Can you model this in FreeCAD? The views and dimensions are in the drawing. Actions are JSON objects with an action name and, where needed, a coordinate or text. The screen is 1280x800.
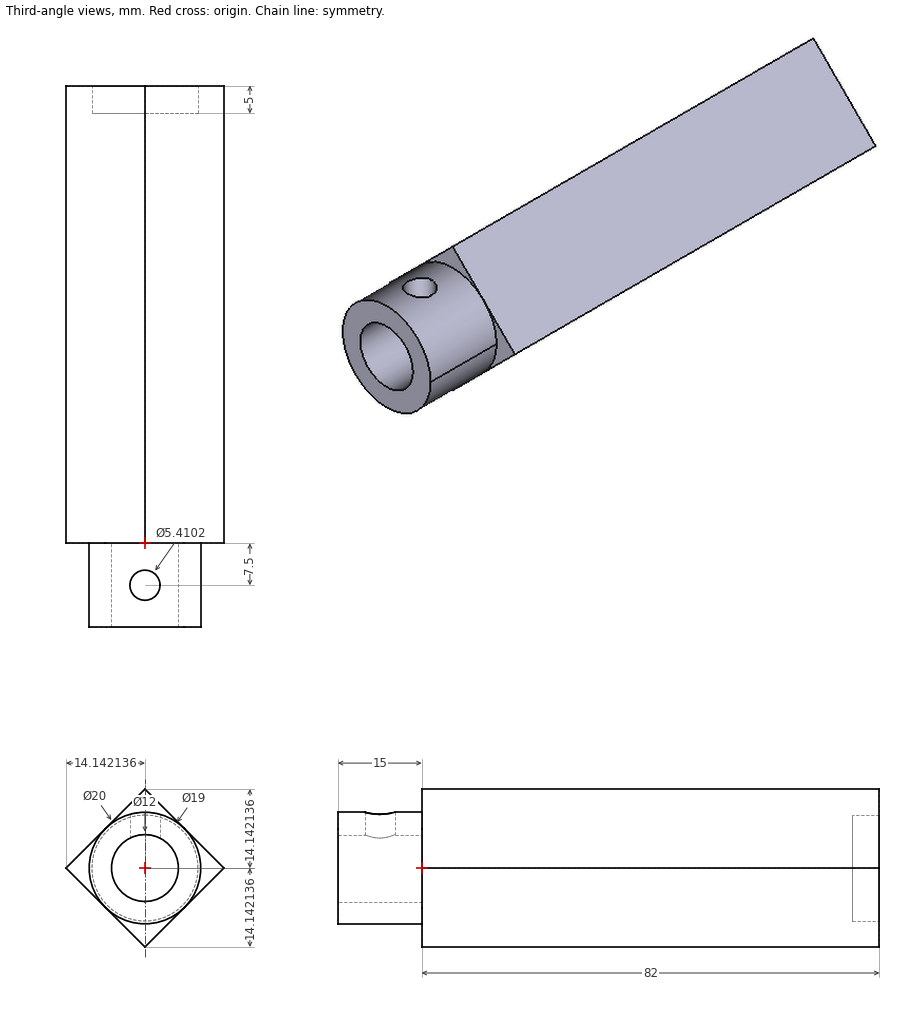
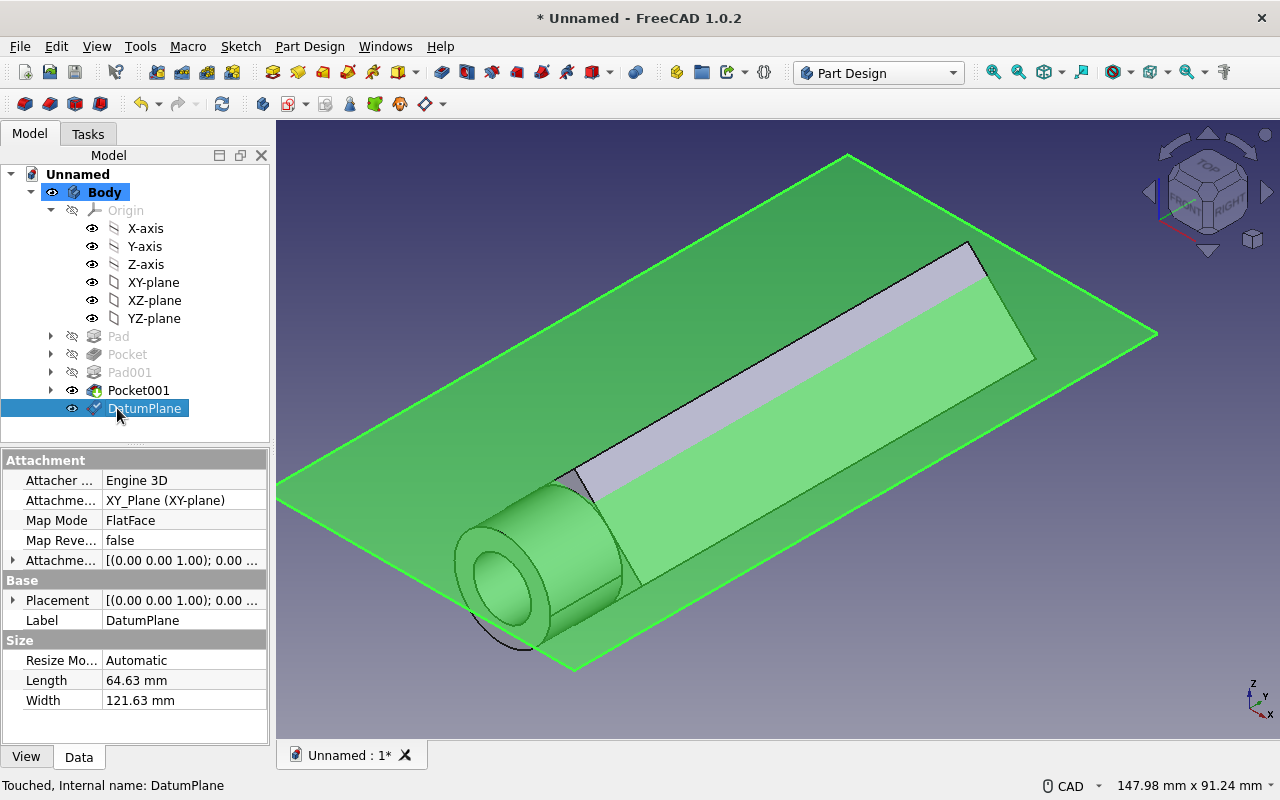
{"action": "left_click", "coordinate": [288, 104]}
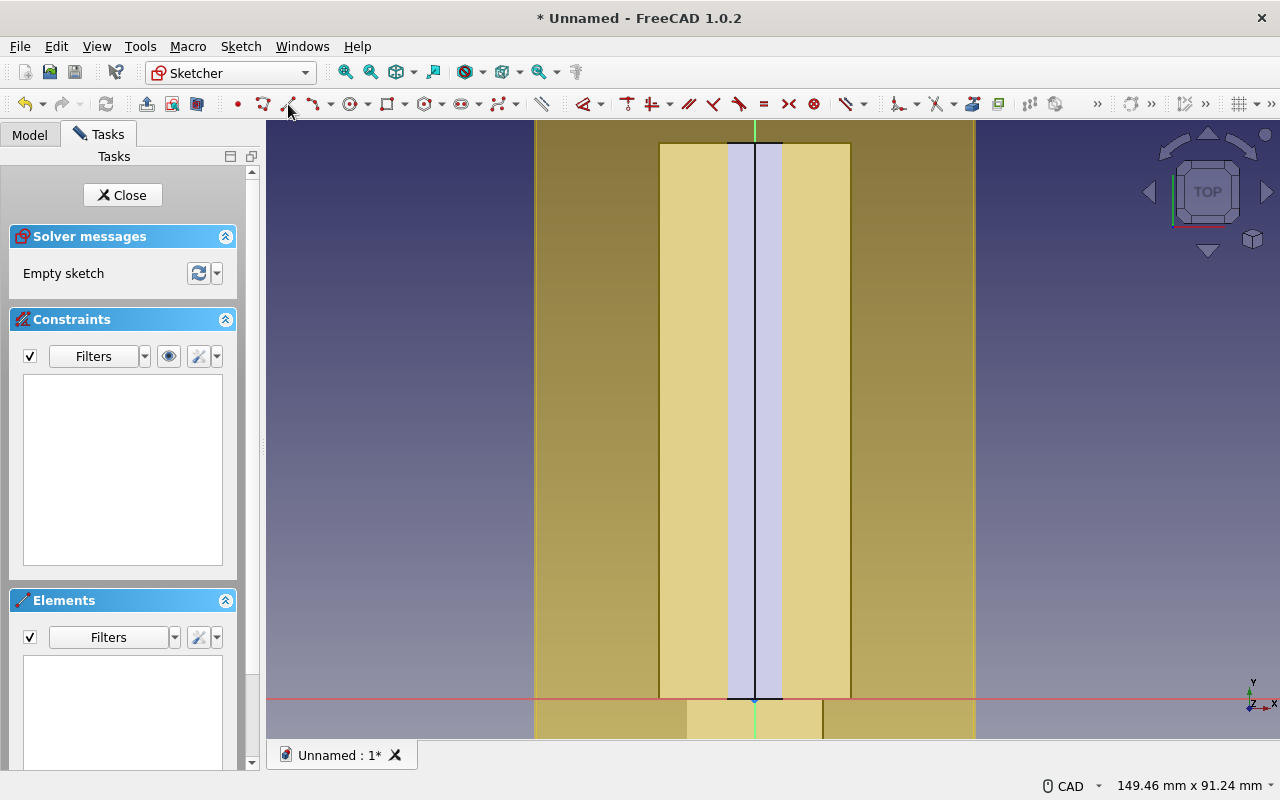
{"action": "key", "text": "q s"}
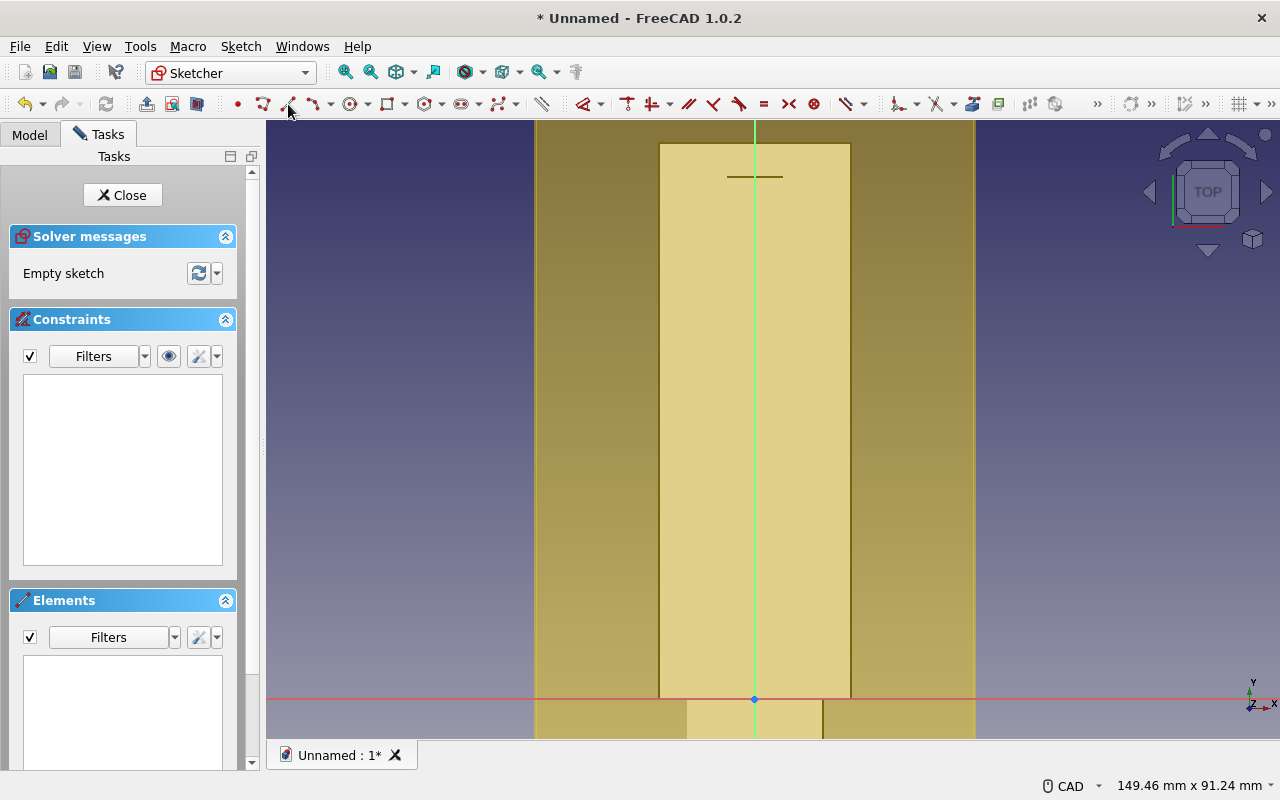
{"action": "scroll", "coordinate": [704, 430], "scroll_direction": "down", "scroll_amount": 5}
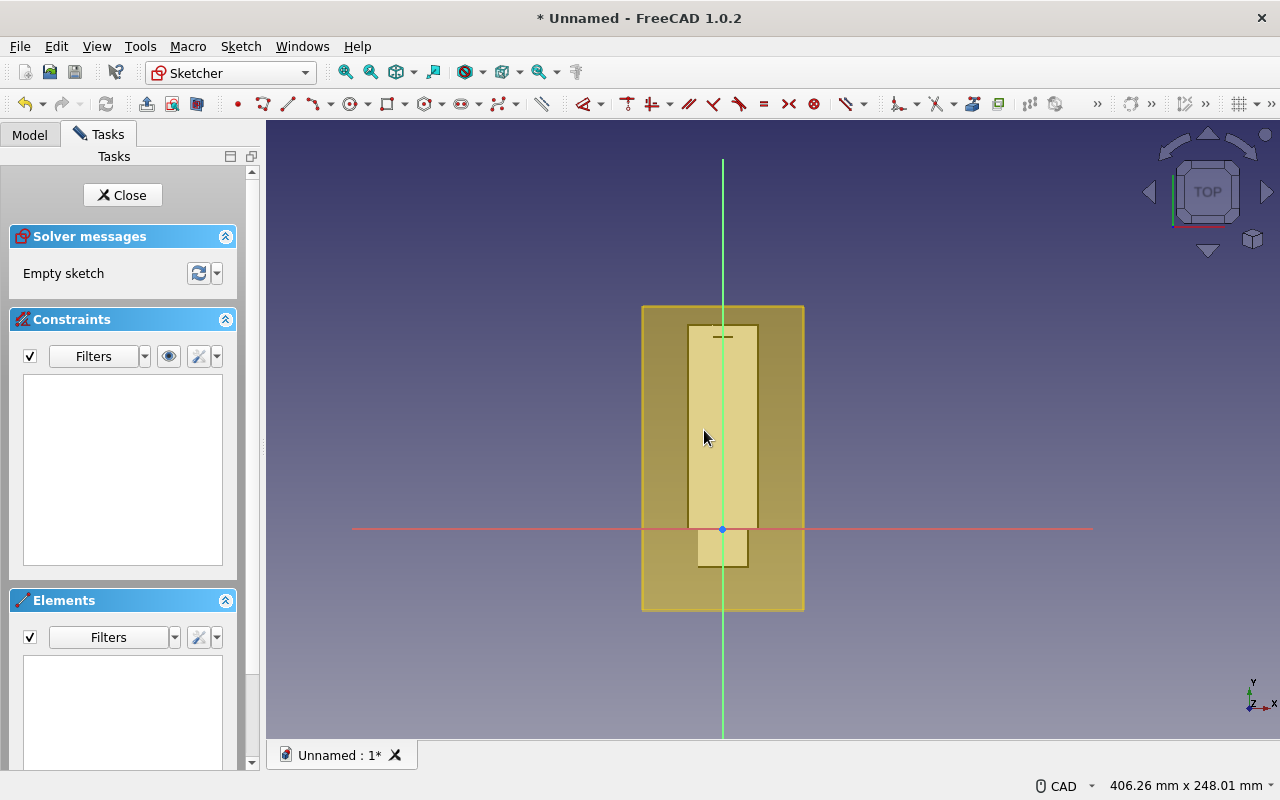
{"action": "scroll", "coordinate": [724, 549], "scroll_direction": "up", "scroll_amount": 14}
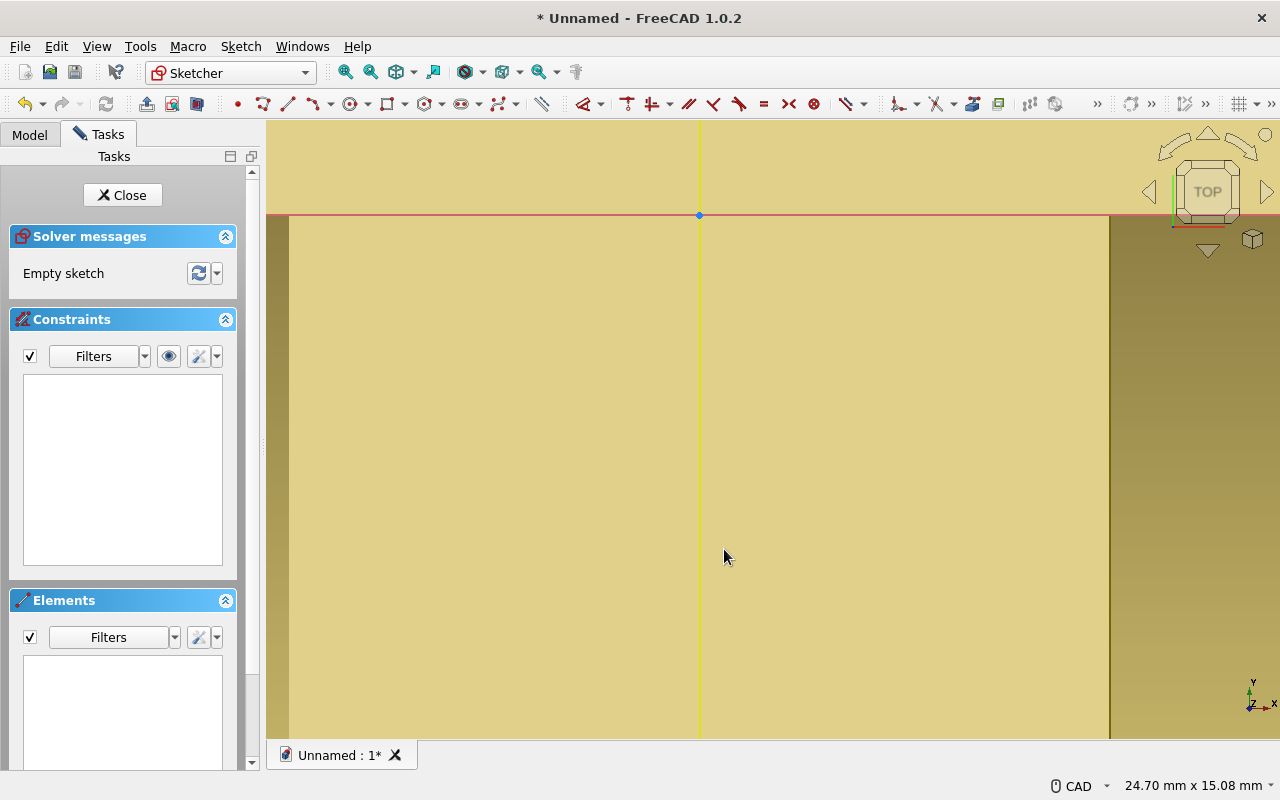
{"action": "key", "text": "g c"}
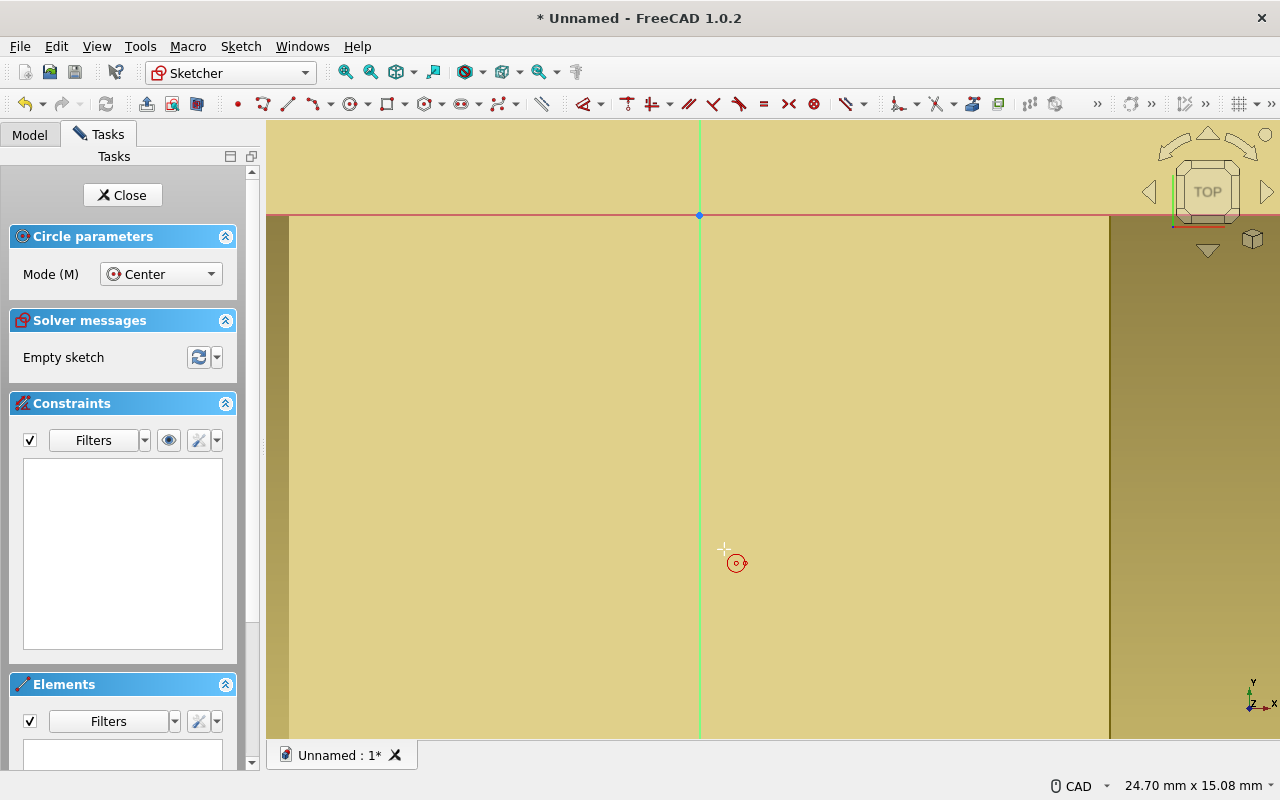
{"action": "left_click", "coordinate": [700, 523]}
{"action": "mouse_move", "coordinate": [778, 445]}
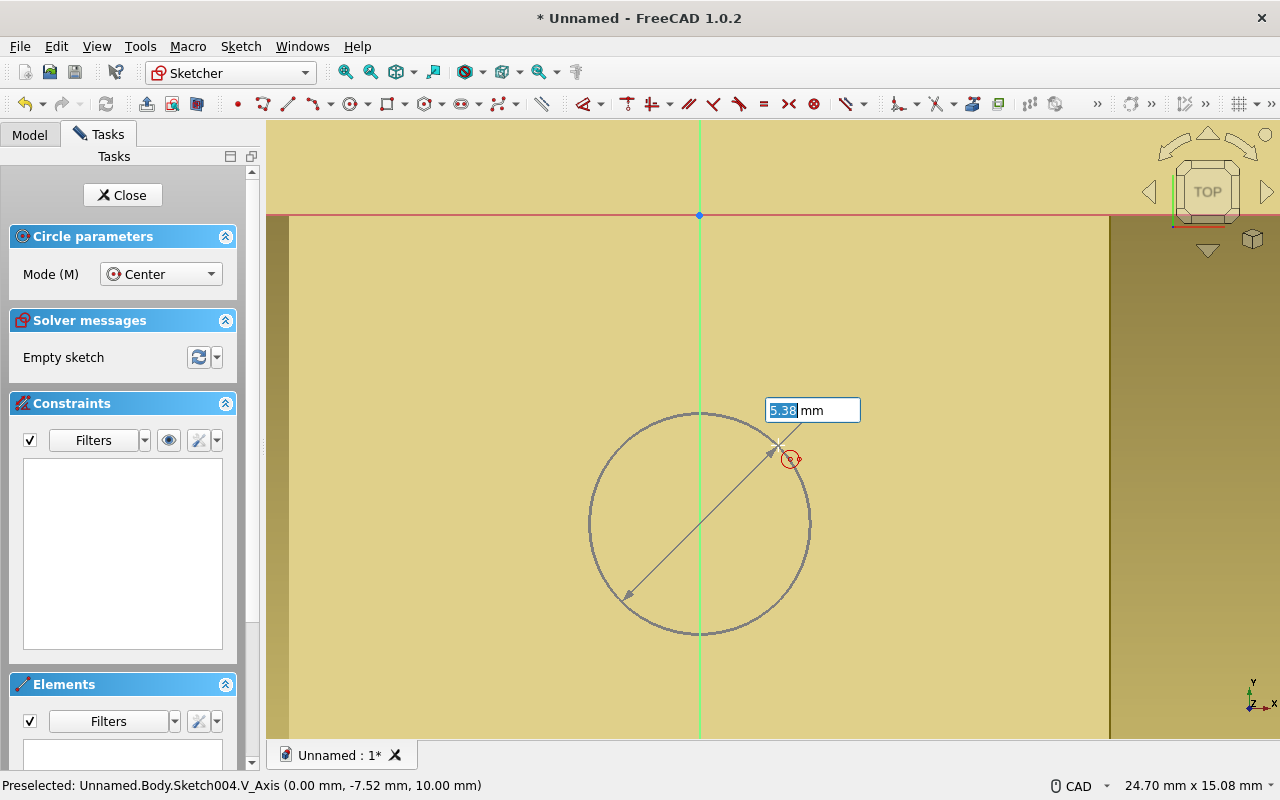
{"action": "type", "text": "5.4102"}
{"action": "key", "text": "Return"}
{"action": "key", "text": "Escape"}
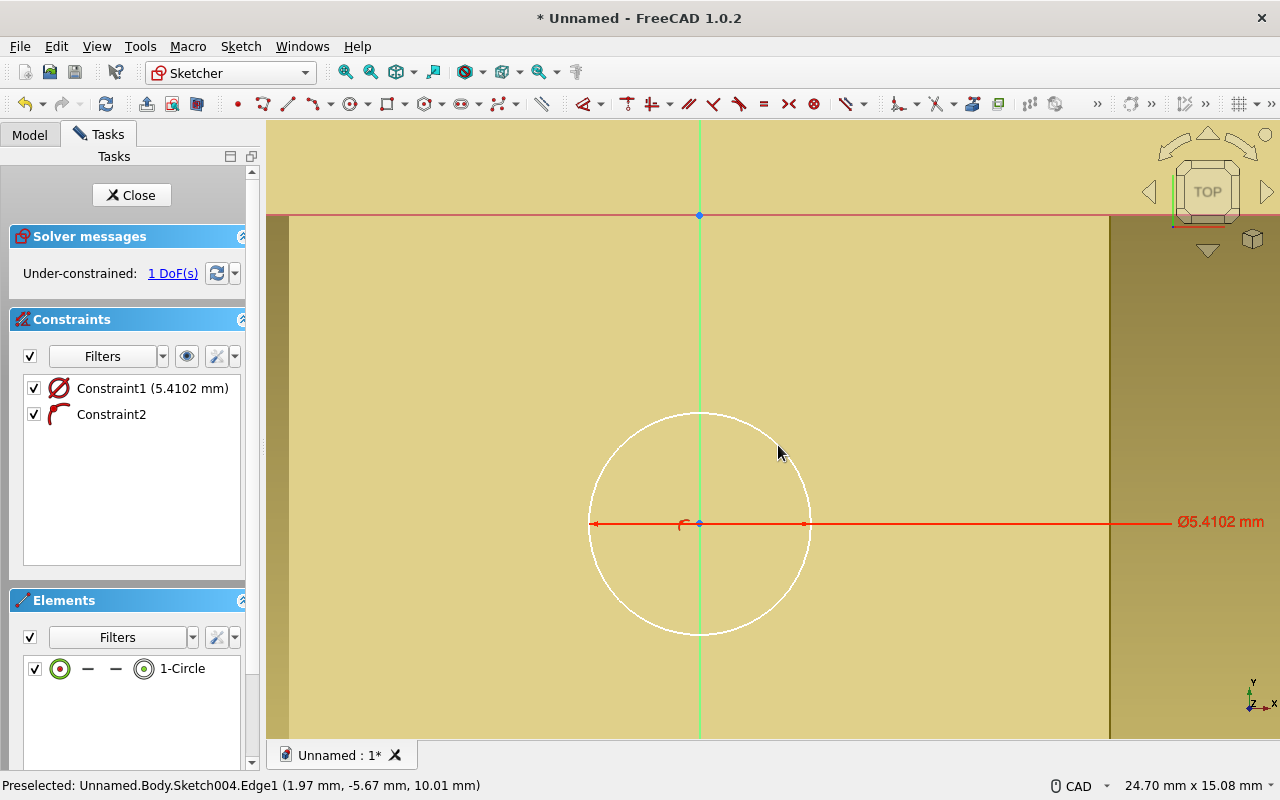
{"action": "key", "text": "d"}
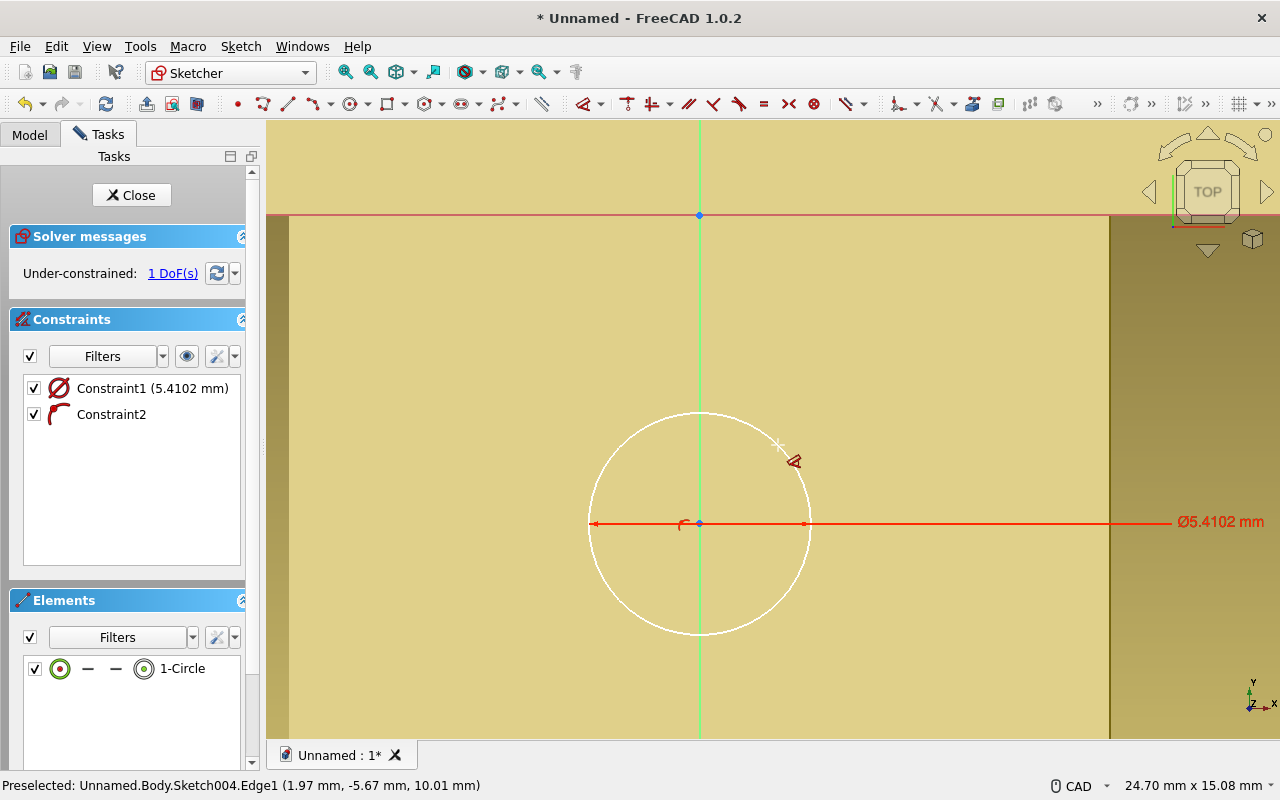
{"action": "left_click", "coordinate": [700, 524]}
{"action": "left_click", "coordinate": [734, 370]}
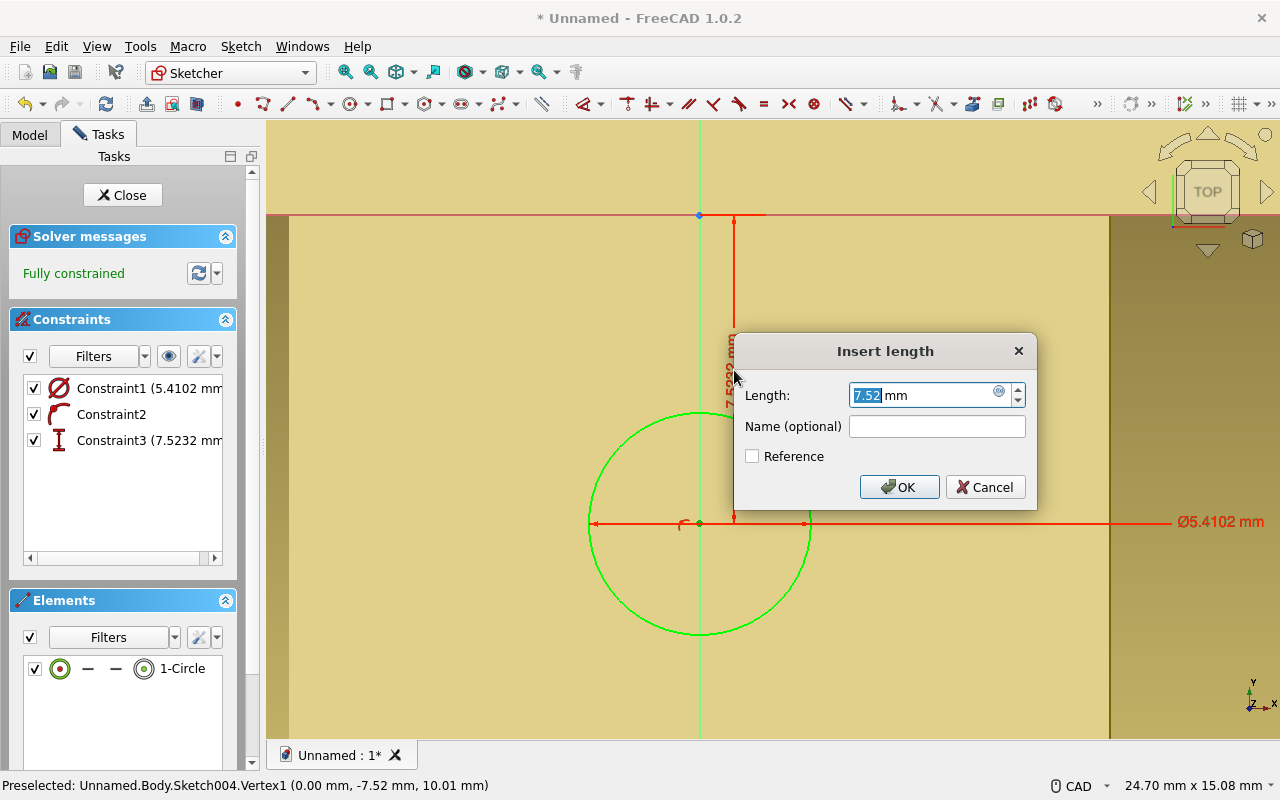
{"action": "type", "text": "7.5"}
{"action": "key", "text": "Return"}
{"action": "key", "text": "Escape"}